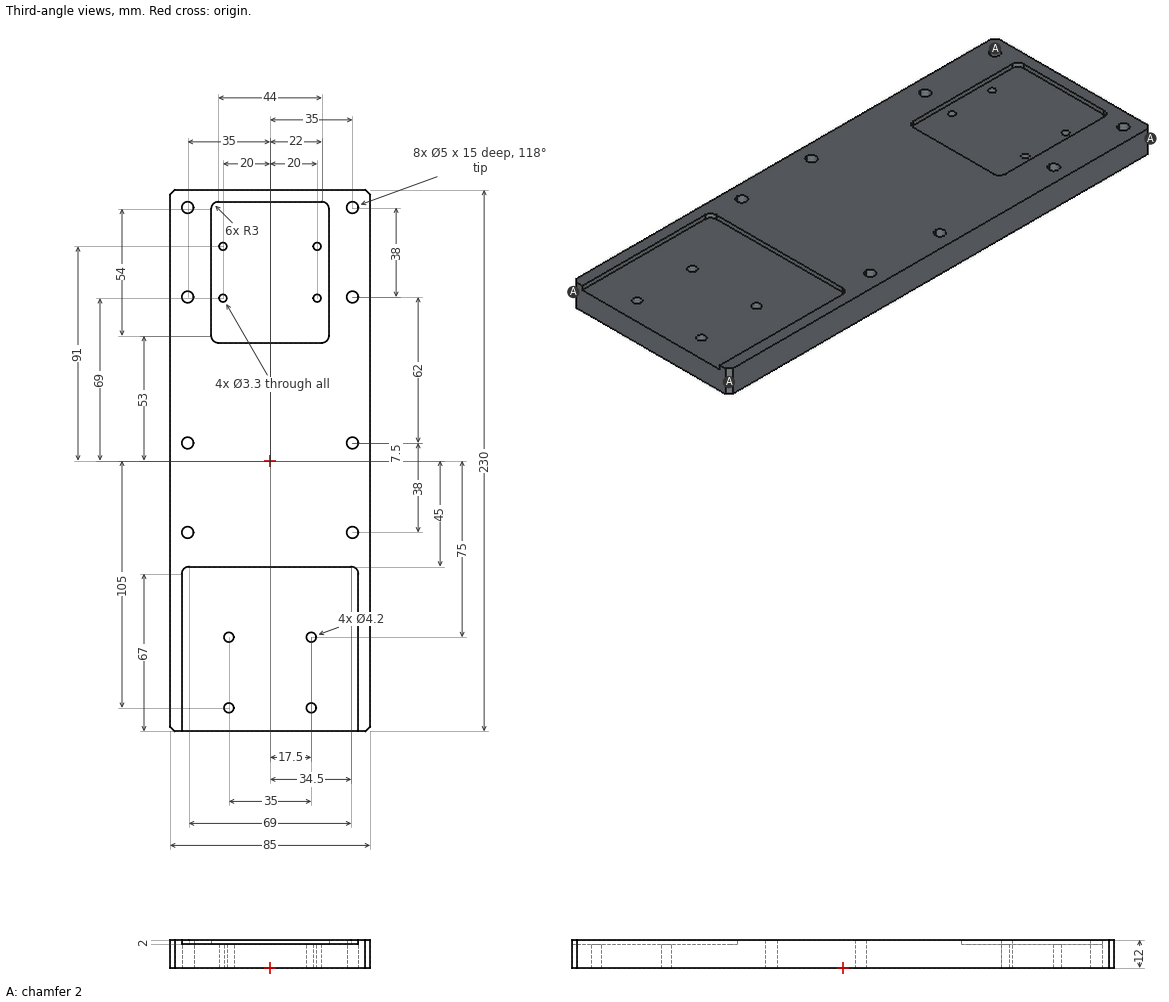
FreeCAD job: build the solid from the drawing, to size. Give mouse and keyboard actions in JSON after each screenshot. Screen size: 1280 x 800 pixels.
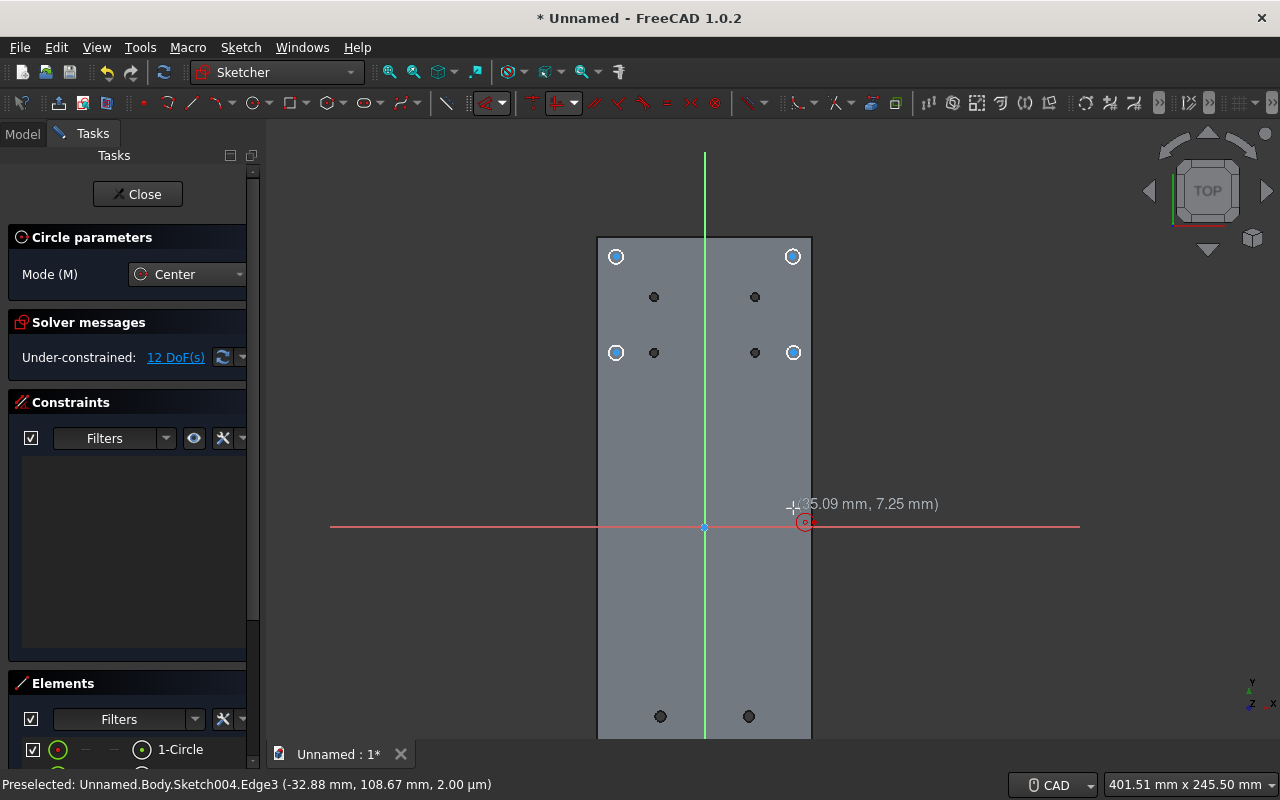
{"action": "left_click", "coordinate": [793, 508]}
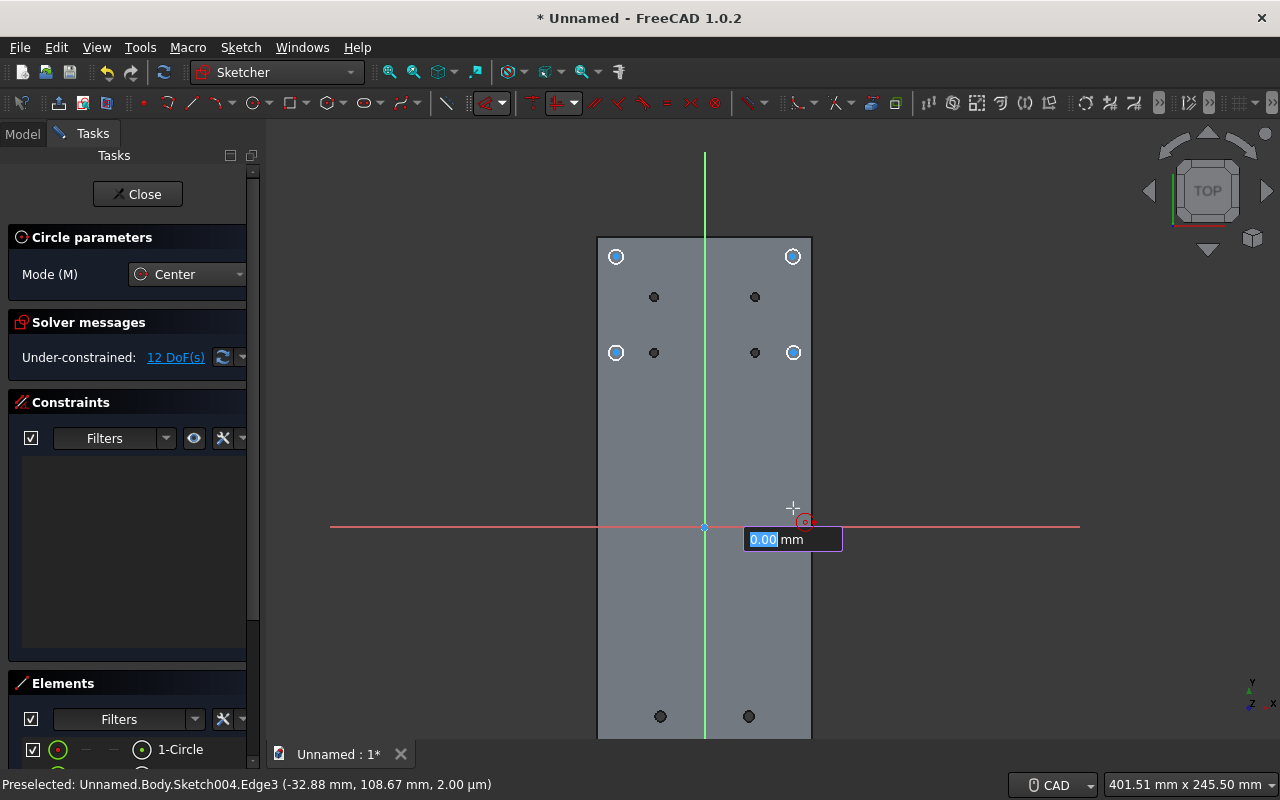
{"action": "scroll", "coordinate": [798, 504], "scroll_direction": "up", "scroll_amount": 5}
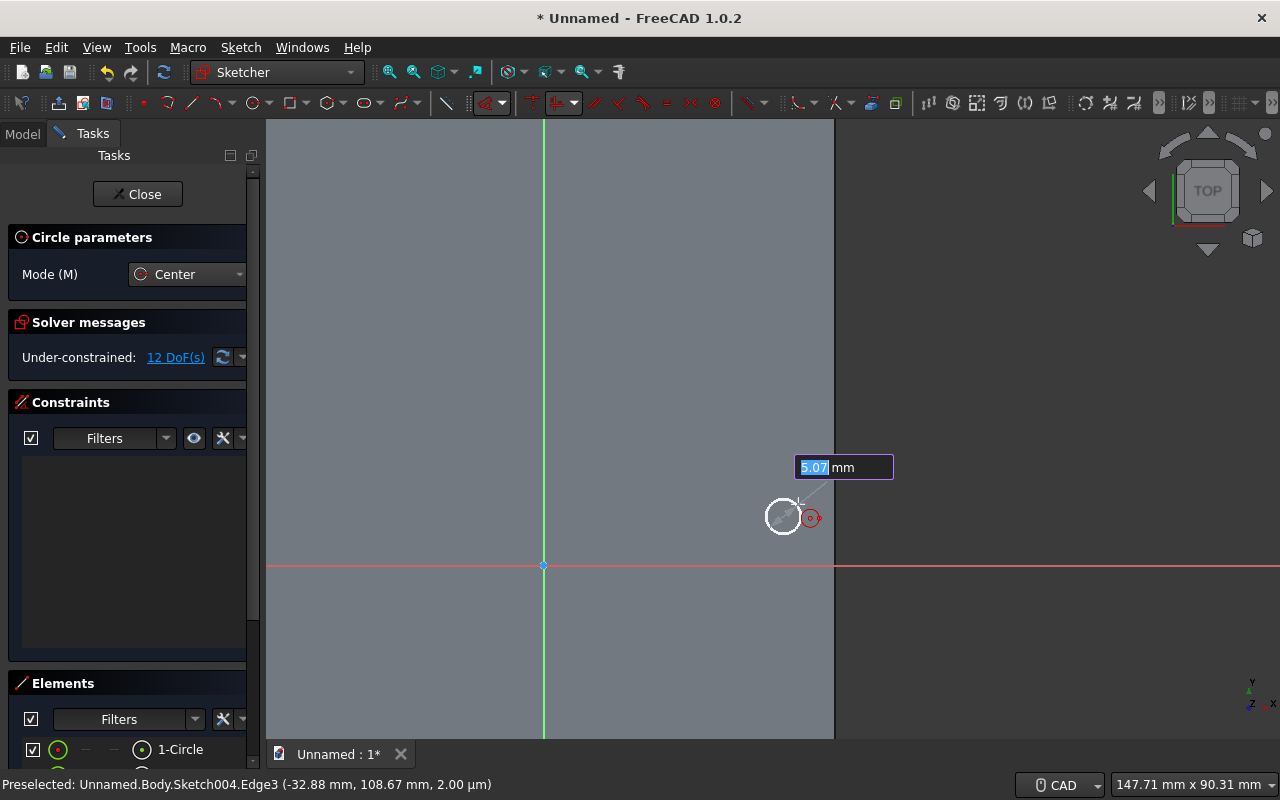
{"action": "left_click", "coordinate": [796, 502]}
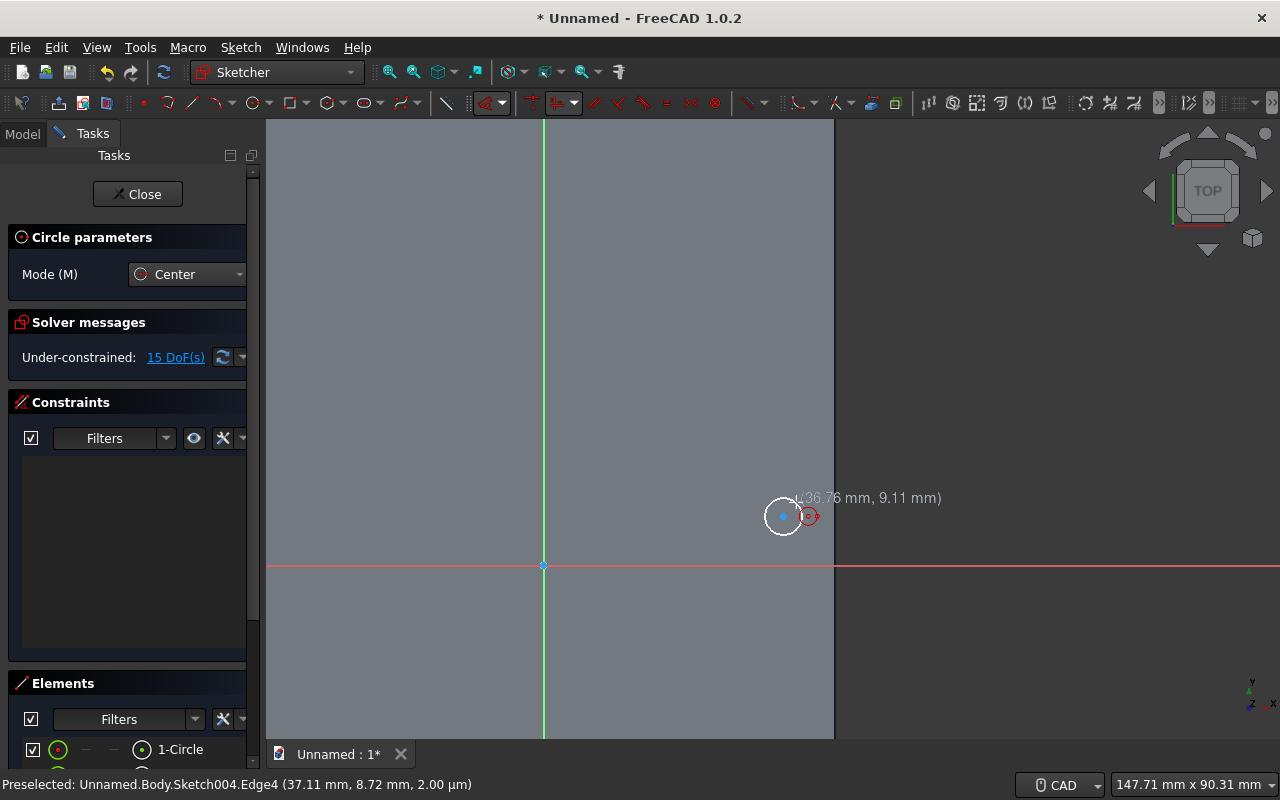
{"action": "scroll", "coordinate": [798, 503], "scroll_direction": "down", "scroll_amount": 5}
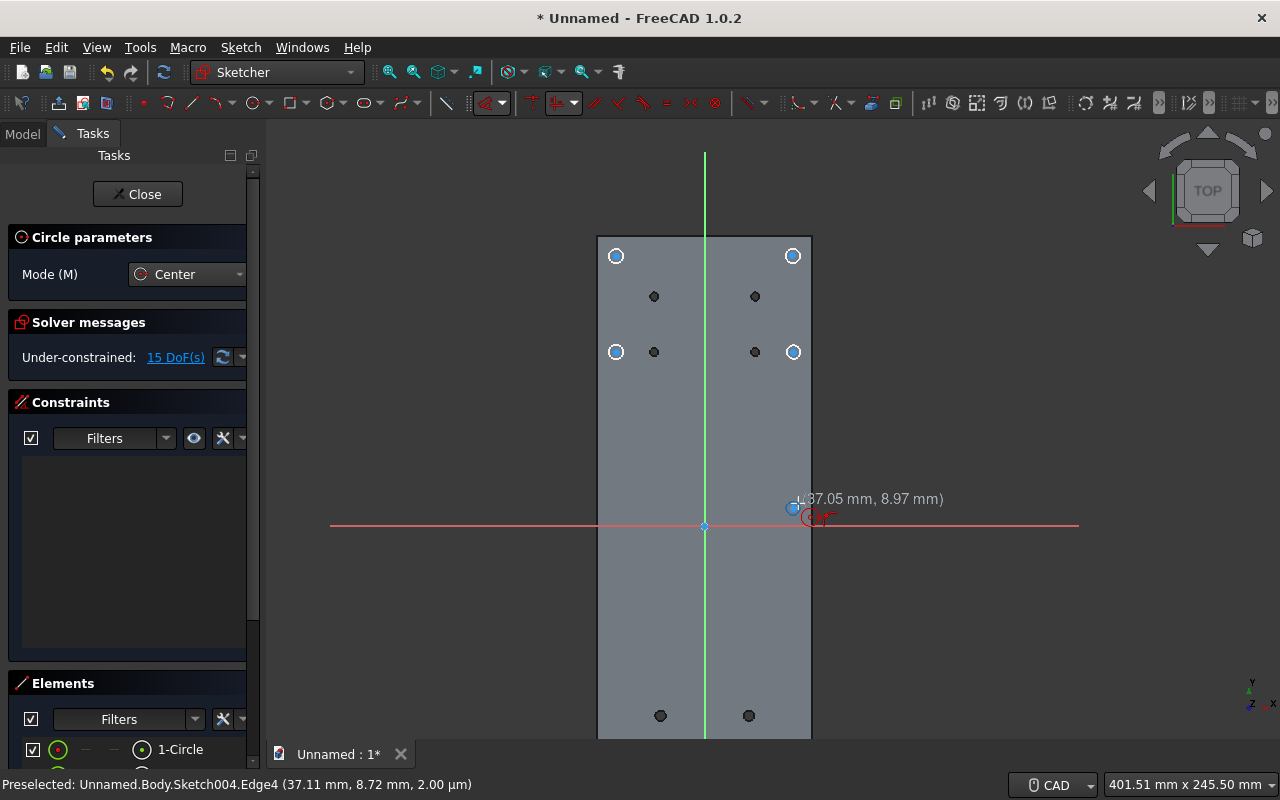
{"action": "scroll", "coordinate": [793, 603], "scroll_direction": "up", "scroll_amount": 7}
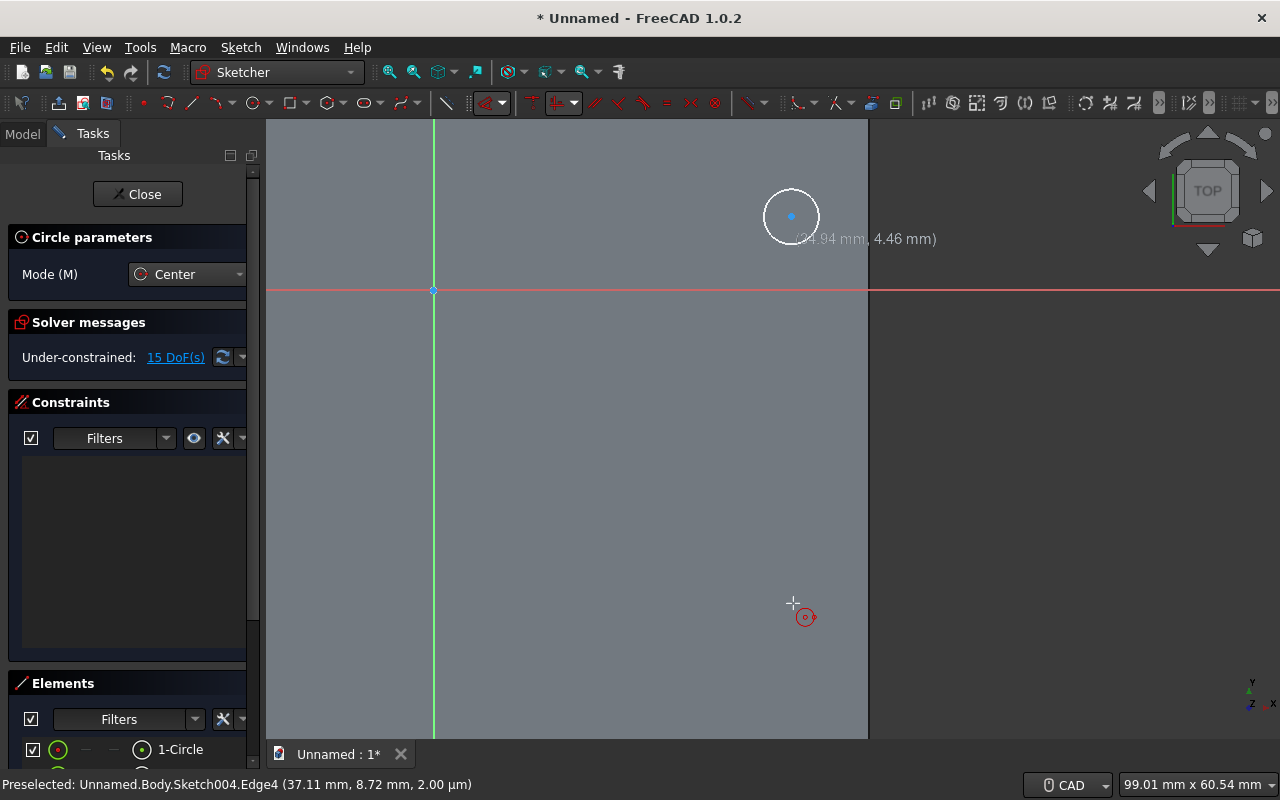
{"action": "scroll", "coordinate": [793, 604], "scroll_direction": "down", "scroll_amount": 7}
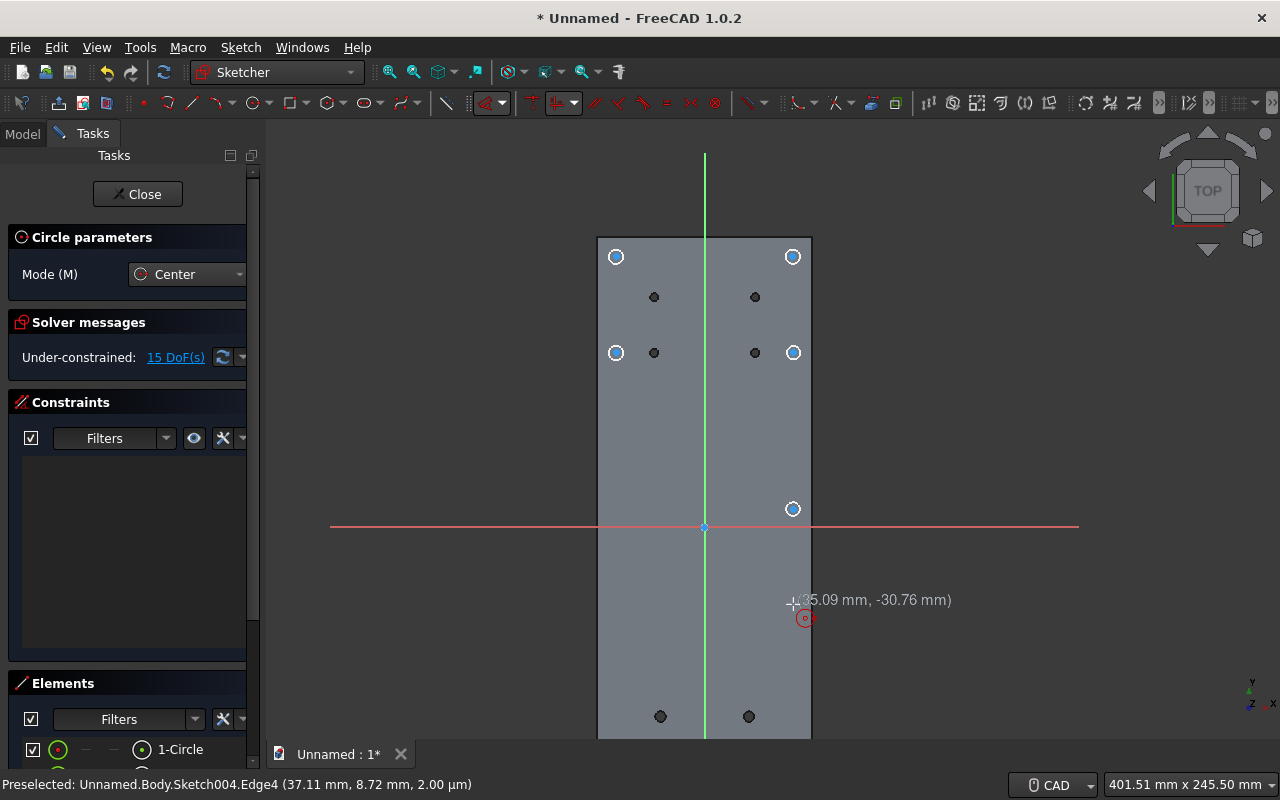
{"action": "left_click", "coordinate": [793, 604]}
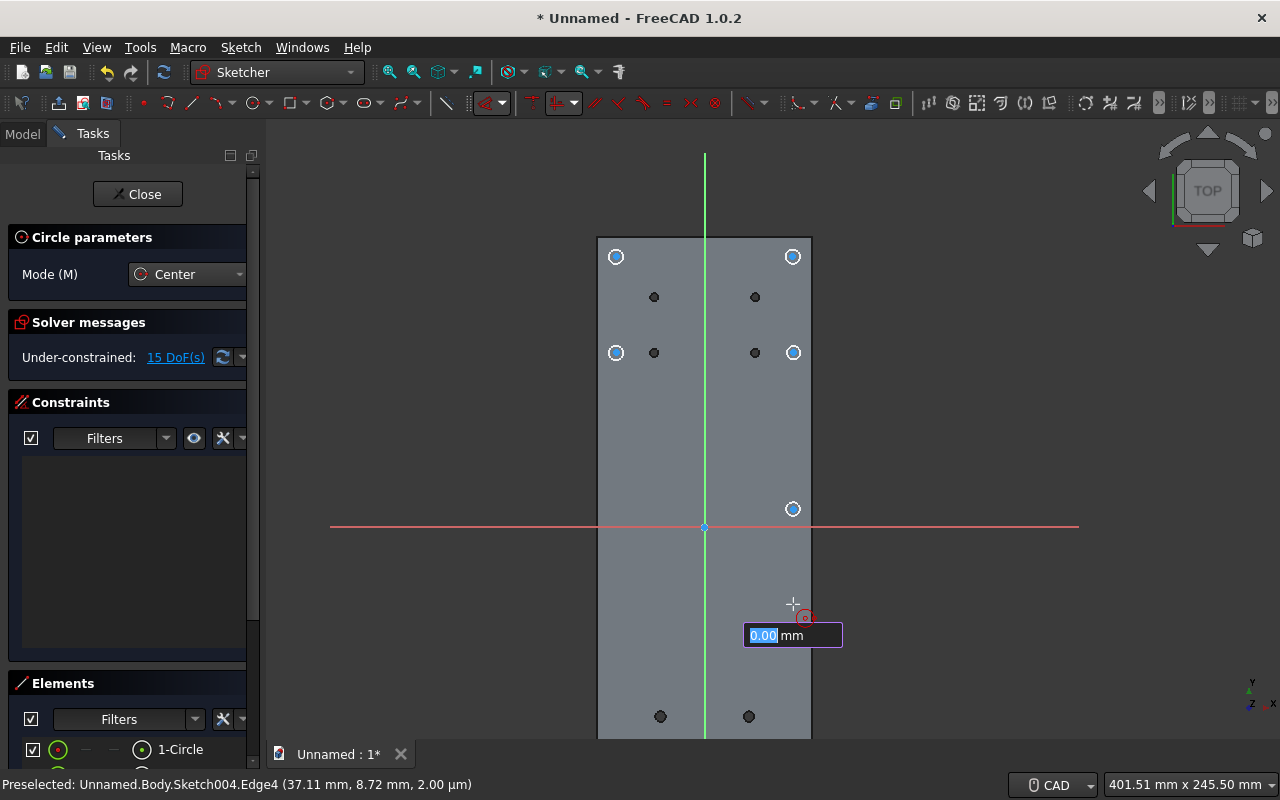
{"action": "scroll", "coordinate": [798, 600], "scroll_direction": "up", "scroll_amount": 5}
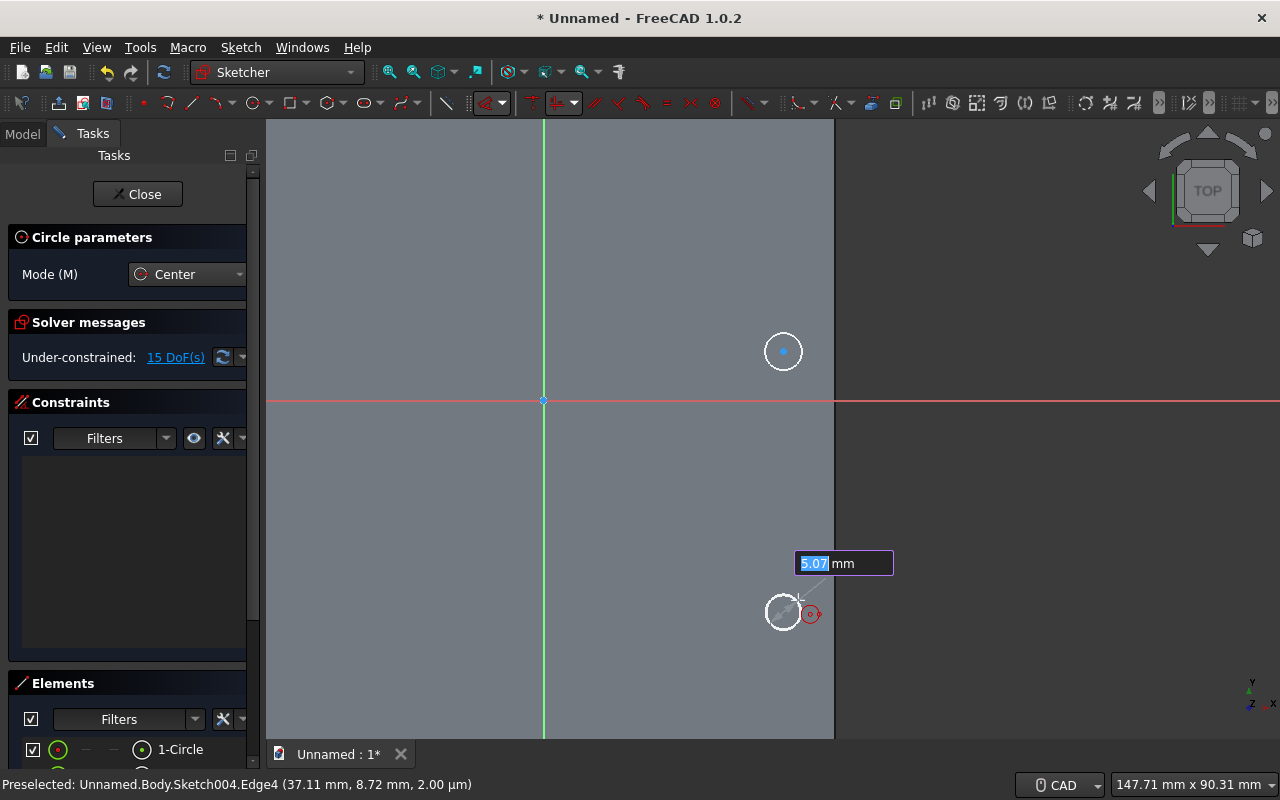
{"action": "left_click", "coordinate": [796, 598]}